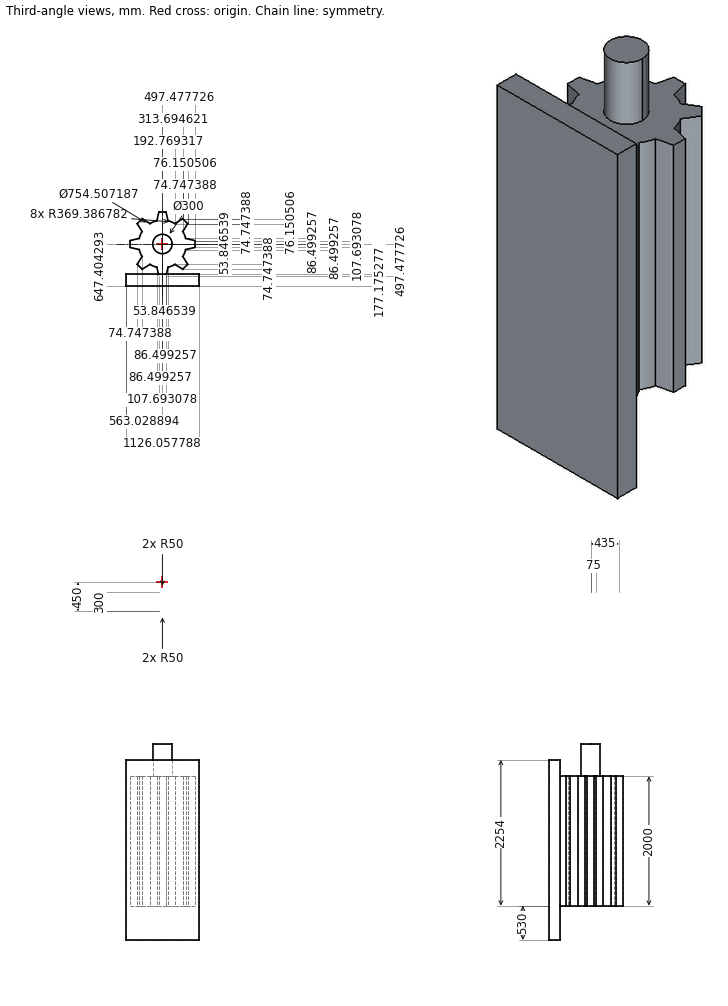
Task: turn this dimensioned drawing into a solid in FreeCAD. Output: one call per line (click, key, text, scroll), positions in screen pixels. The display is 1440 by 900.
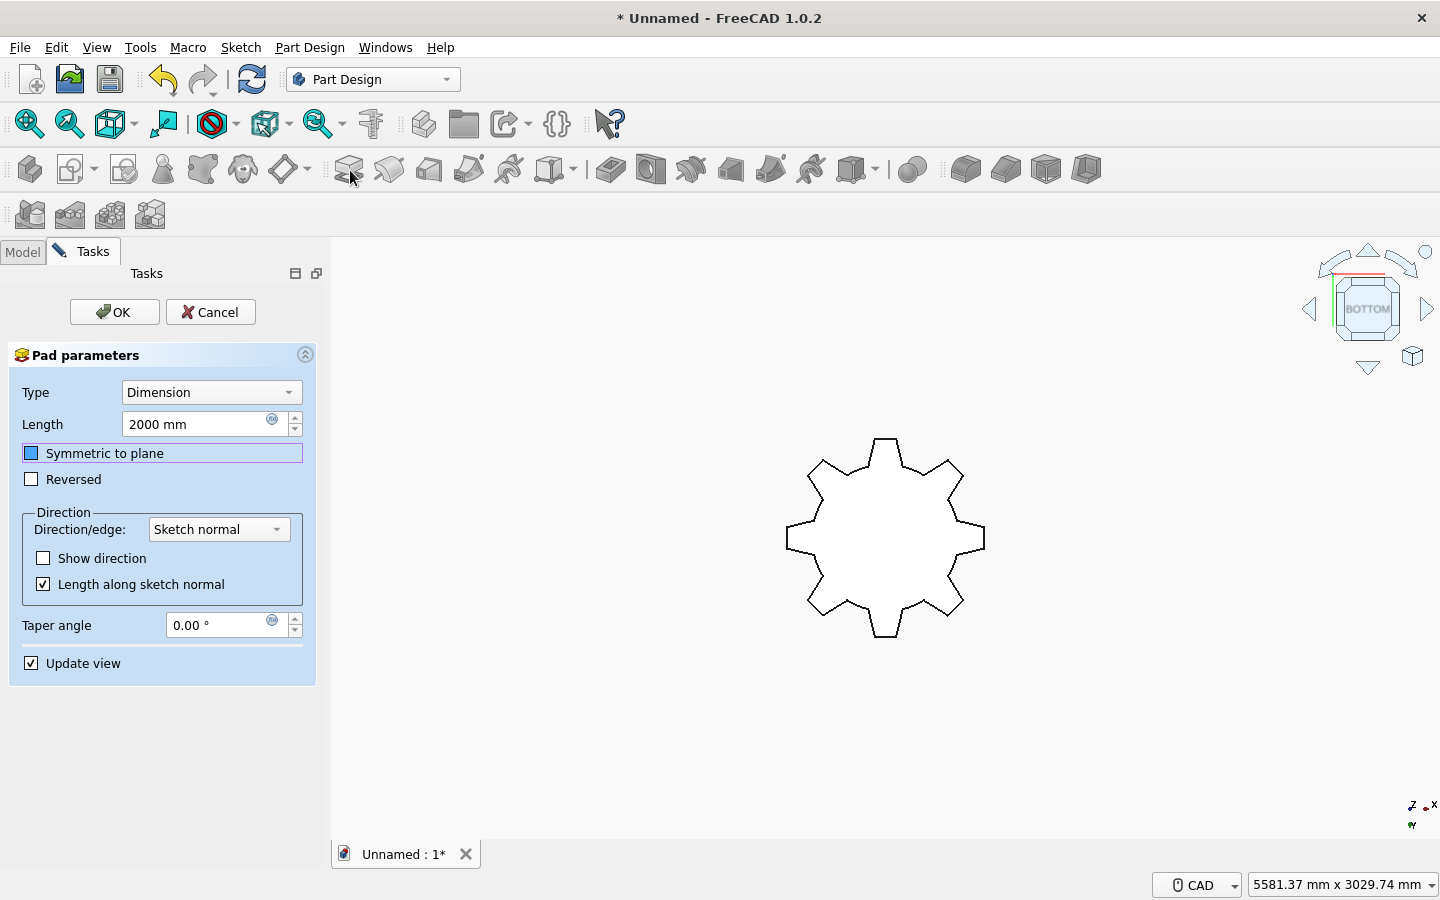
click(115, 312)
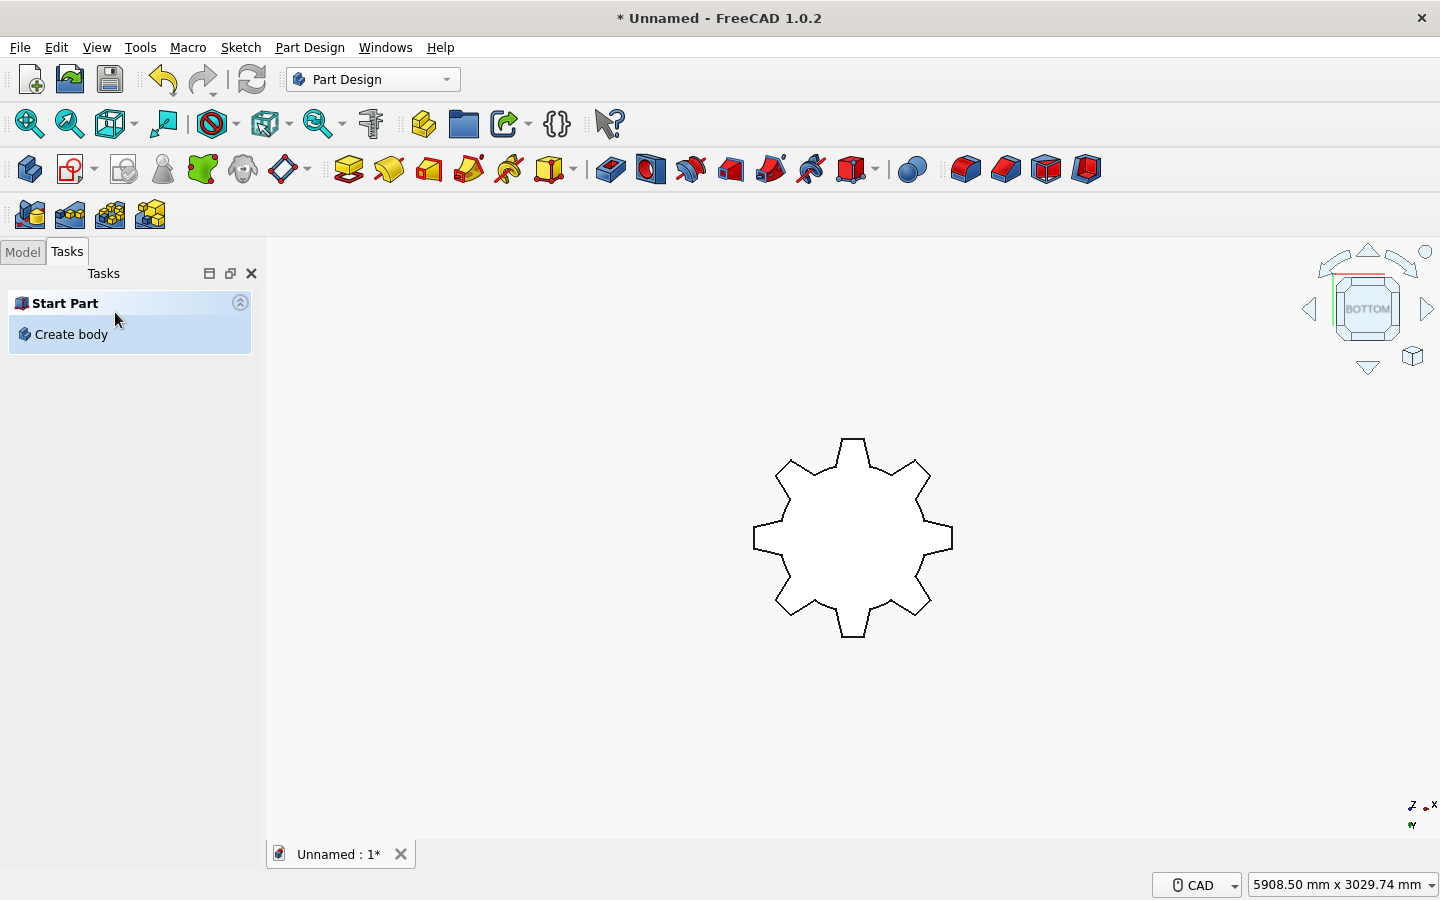
click(30, 124)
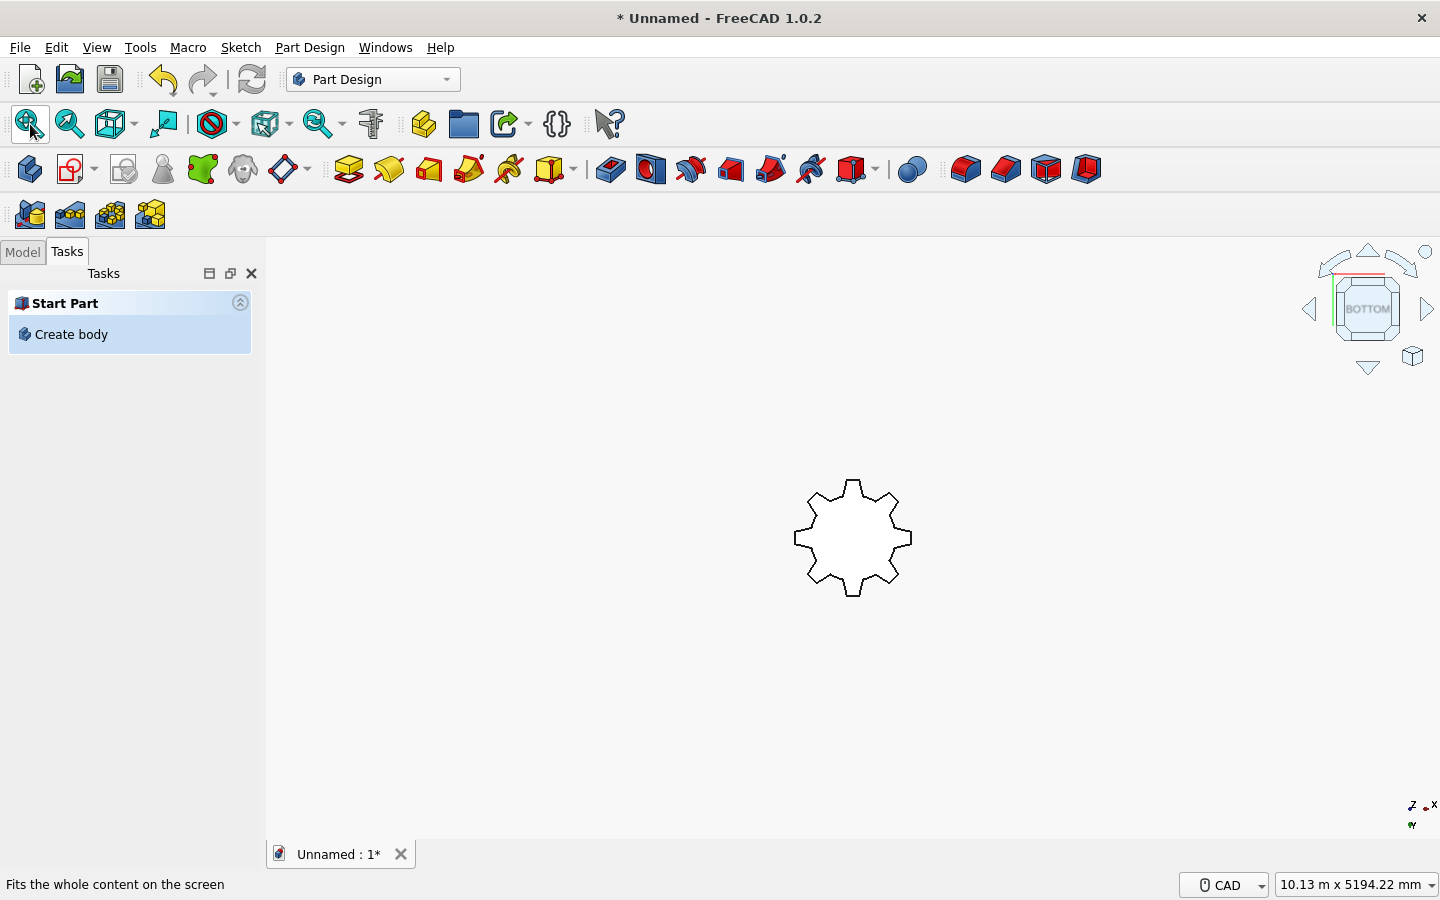
click(853, 537)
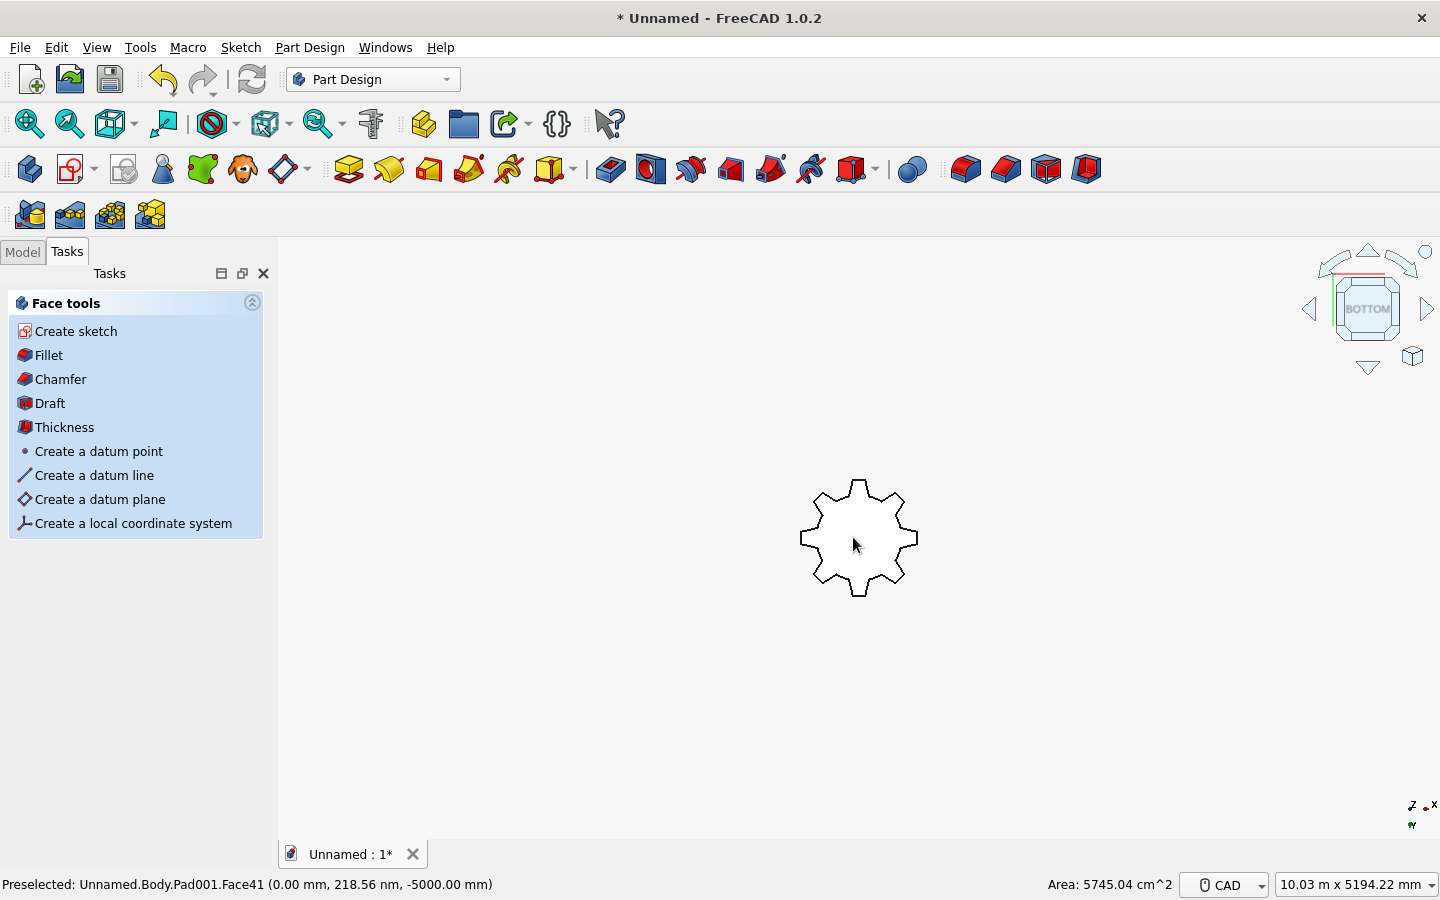
click(70, 170)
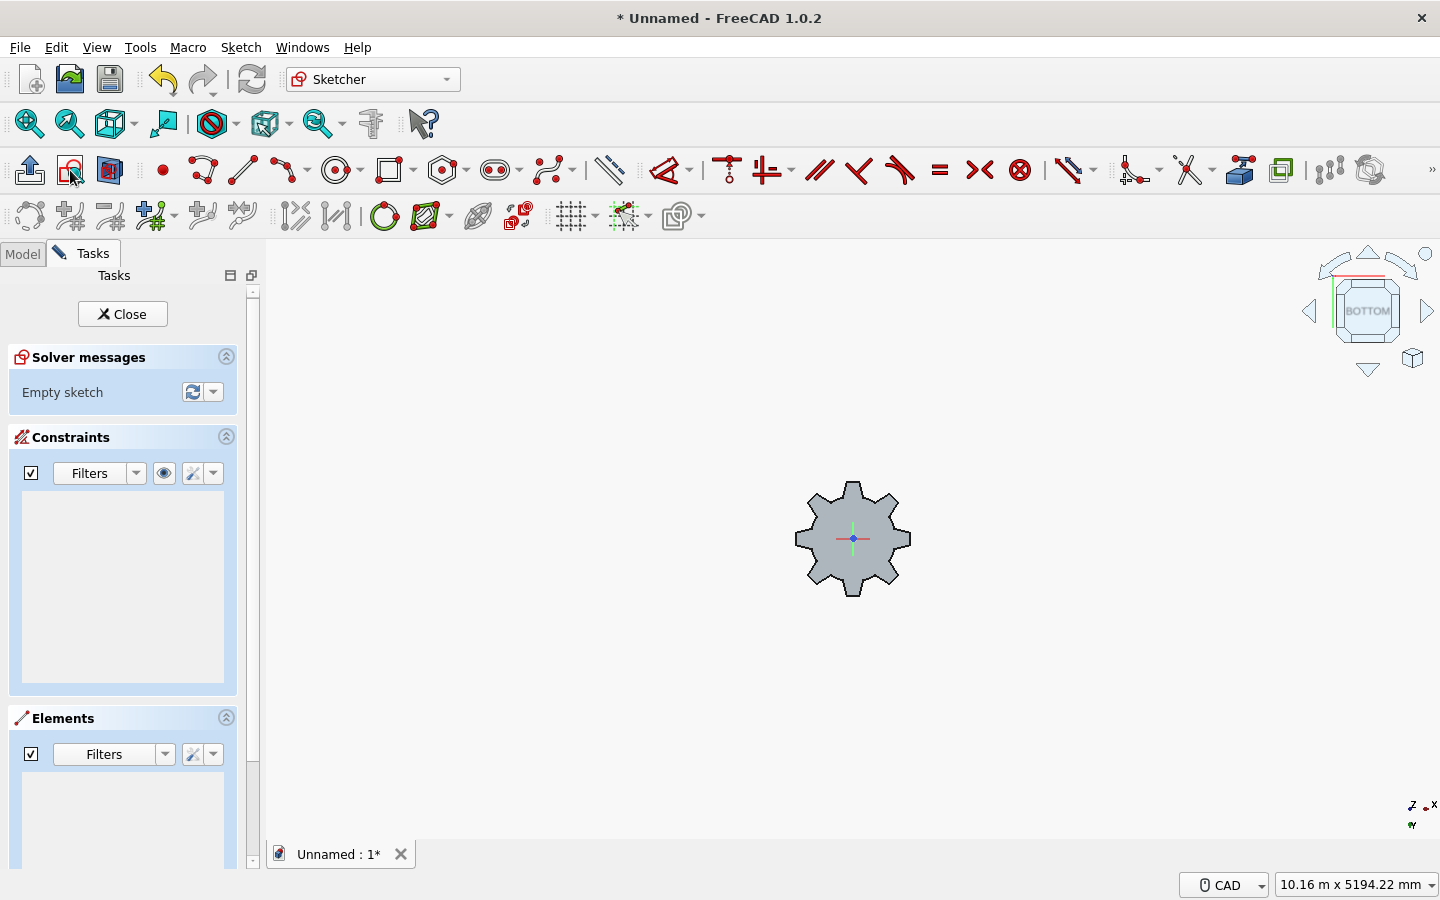
scroll(870, 492, up, 8)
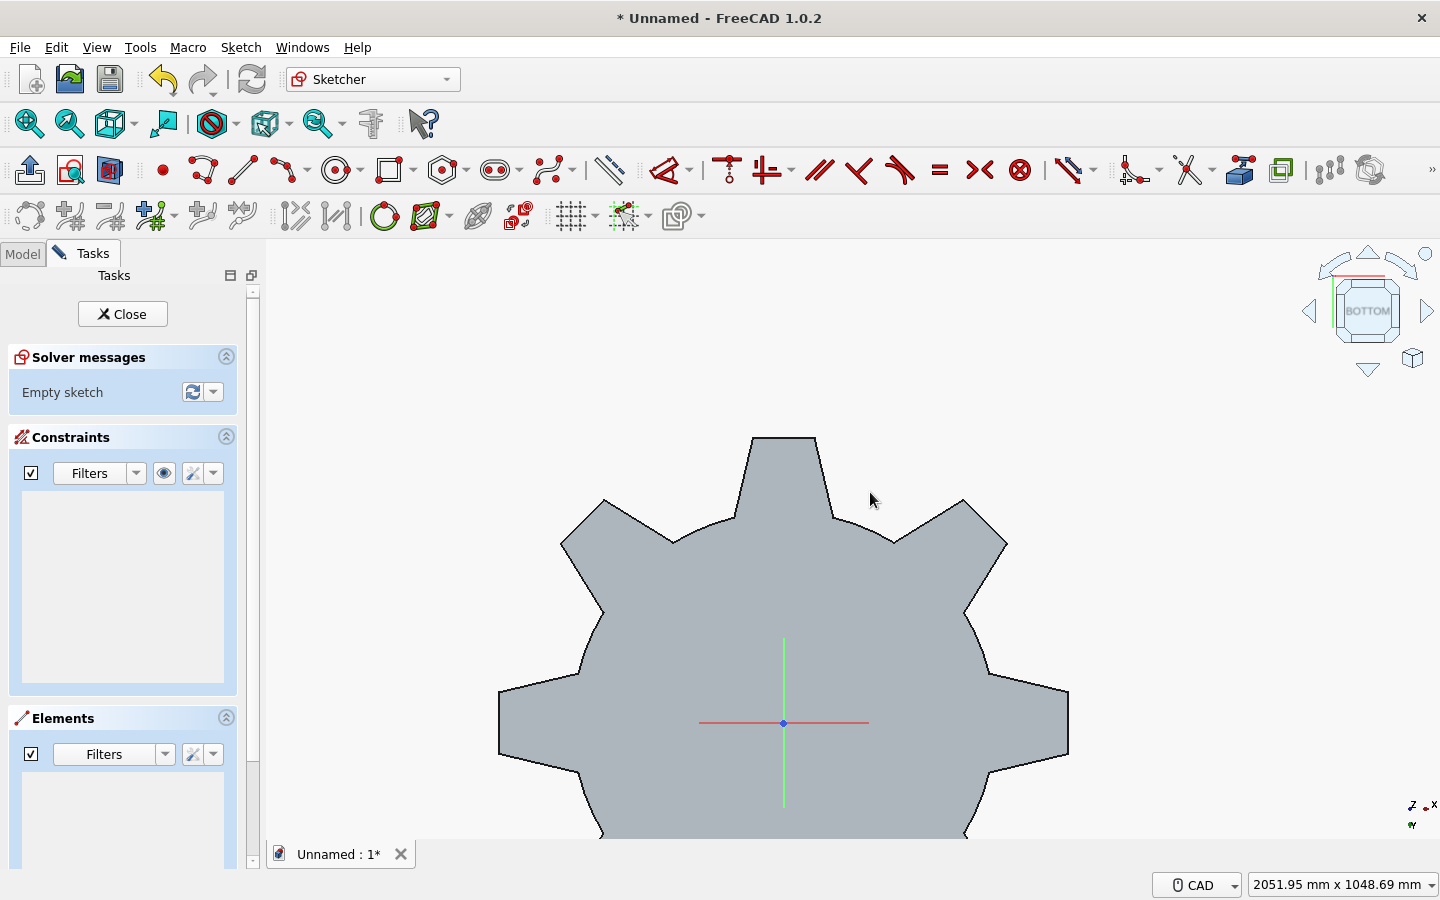
click(390, 170)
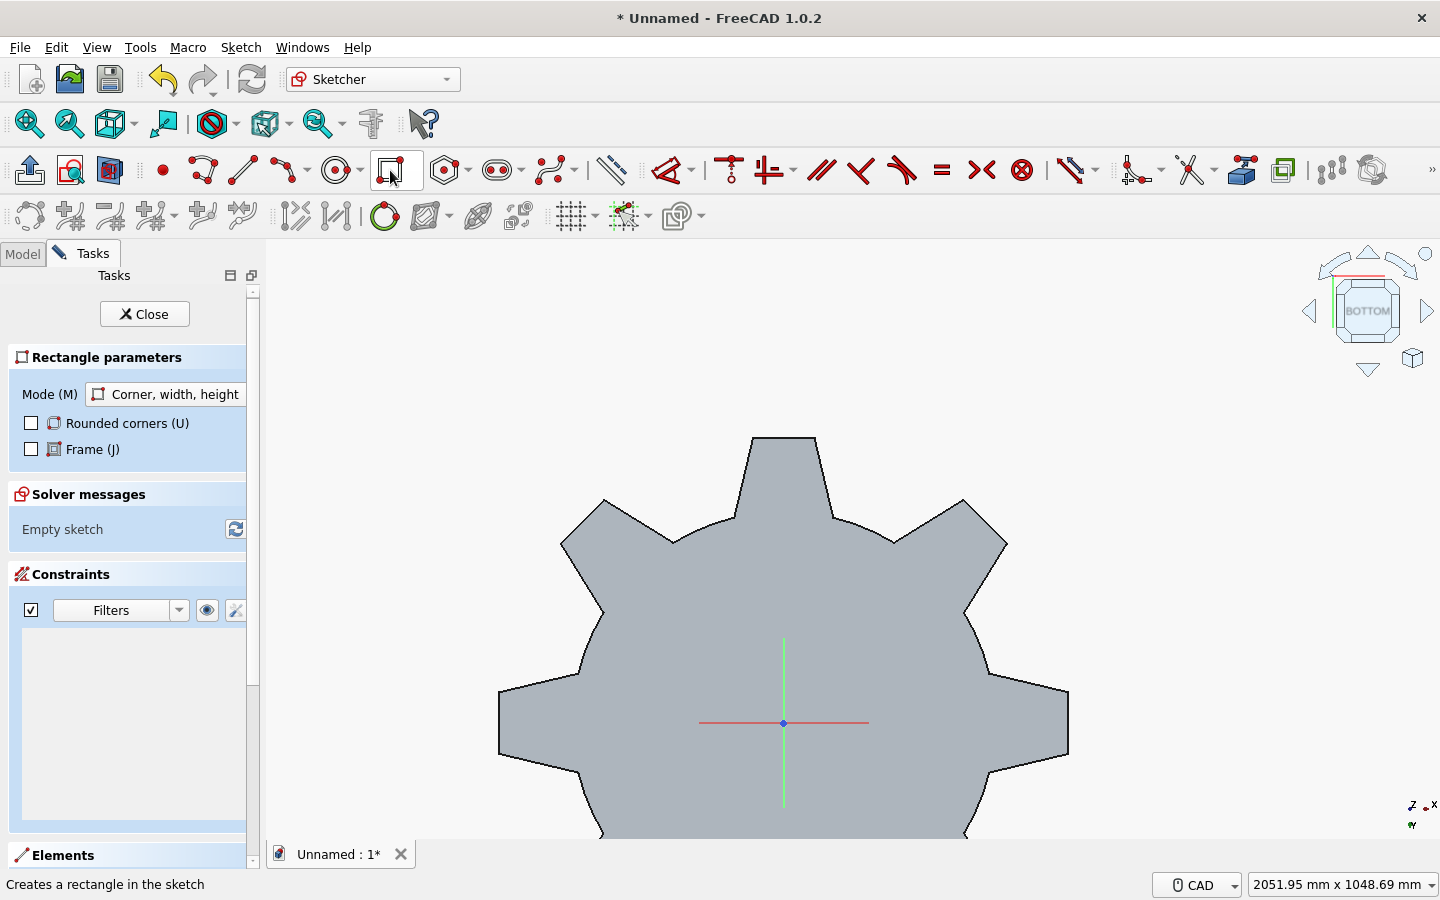
click(462, 353)
move(1106, 454)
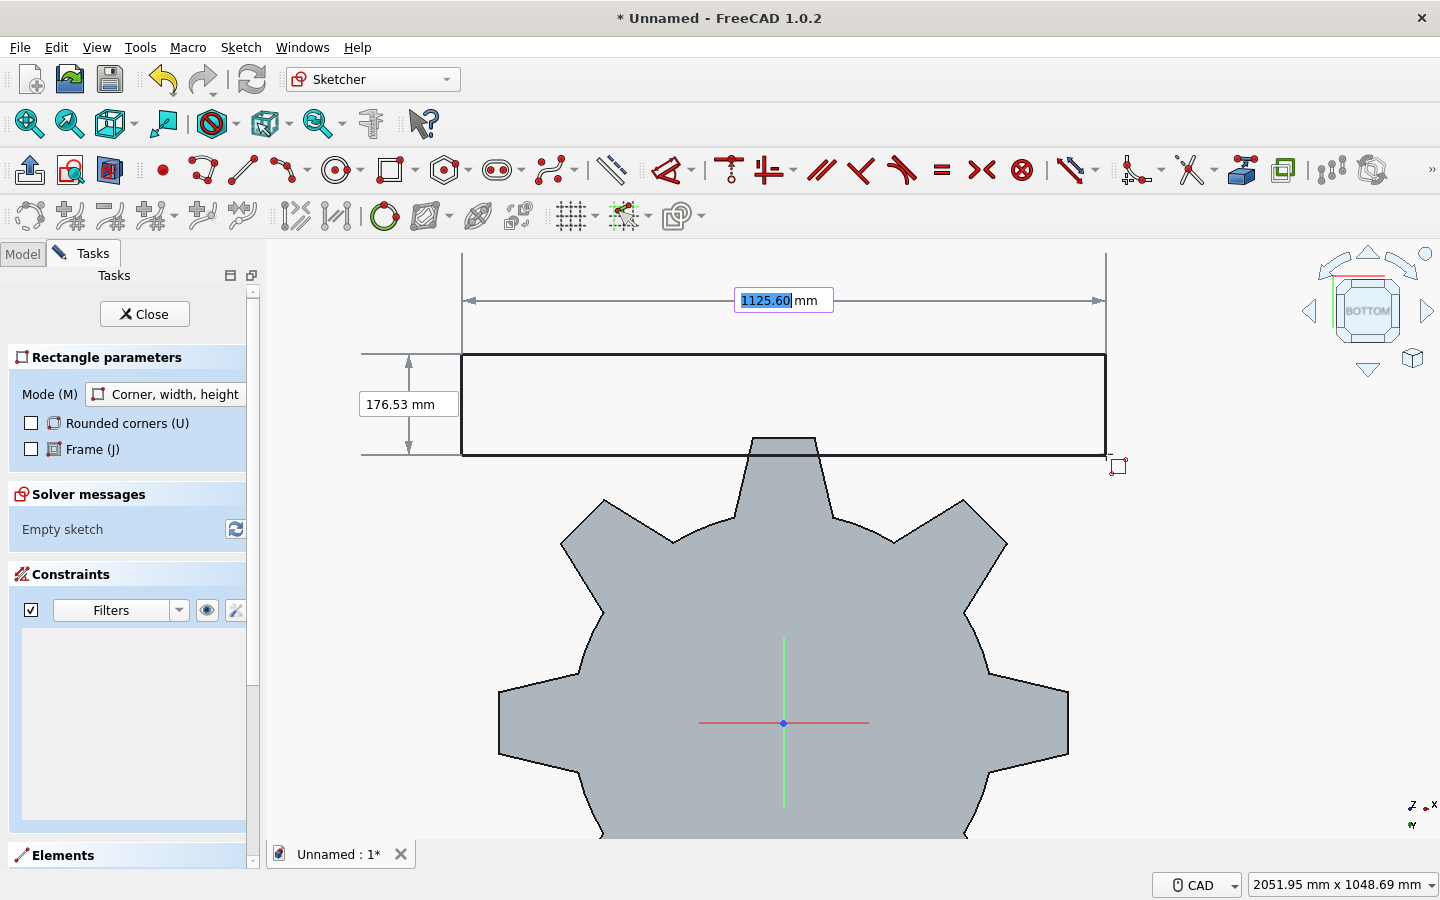
text(1126.057788)
key(Tab)
text(177.175277)
key(Return)
key(Escape)